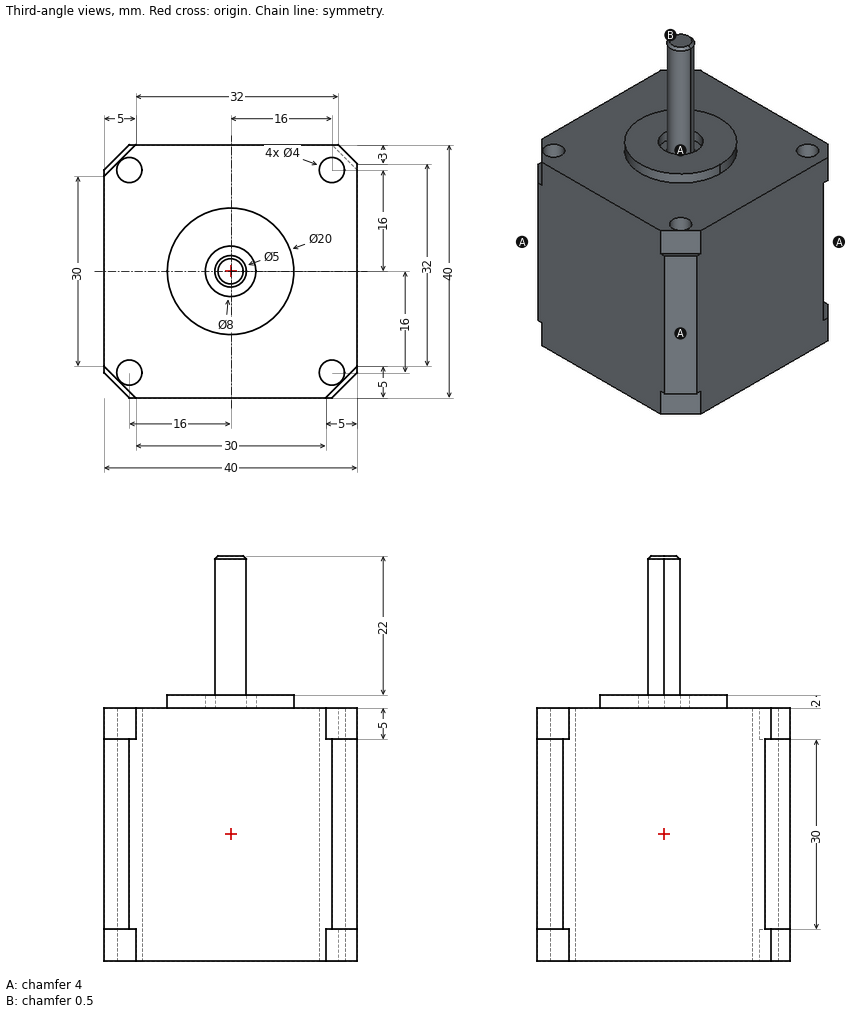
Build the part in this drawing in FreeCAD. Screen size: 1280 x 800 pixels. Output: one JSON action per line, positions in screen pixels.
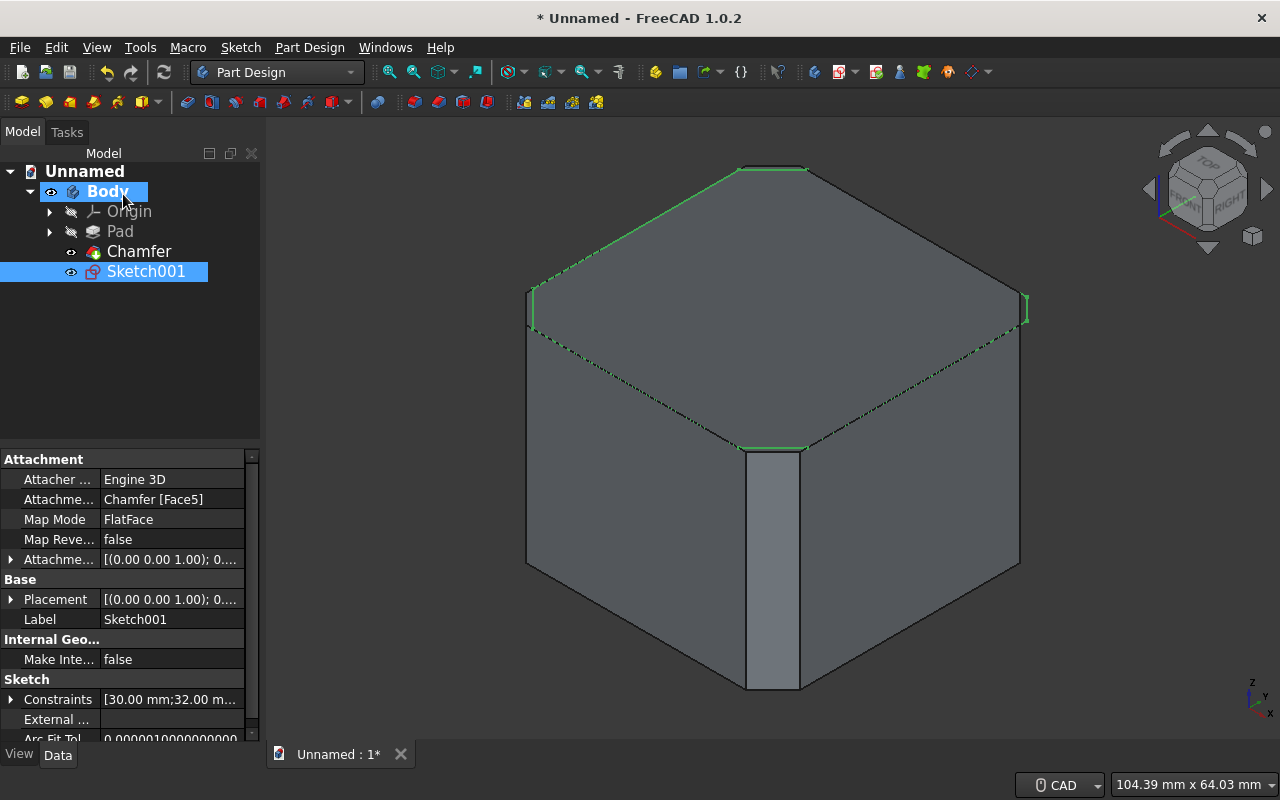
{"action": "left_click", "coordinate": [22, 102]}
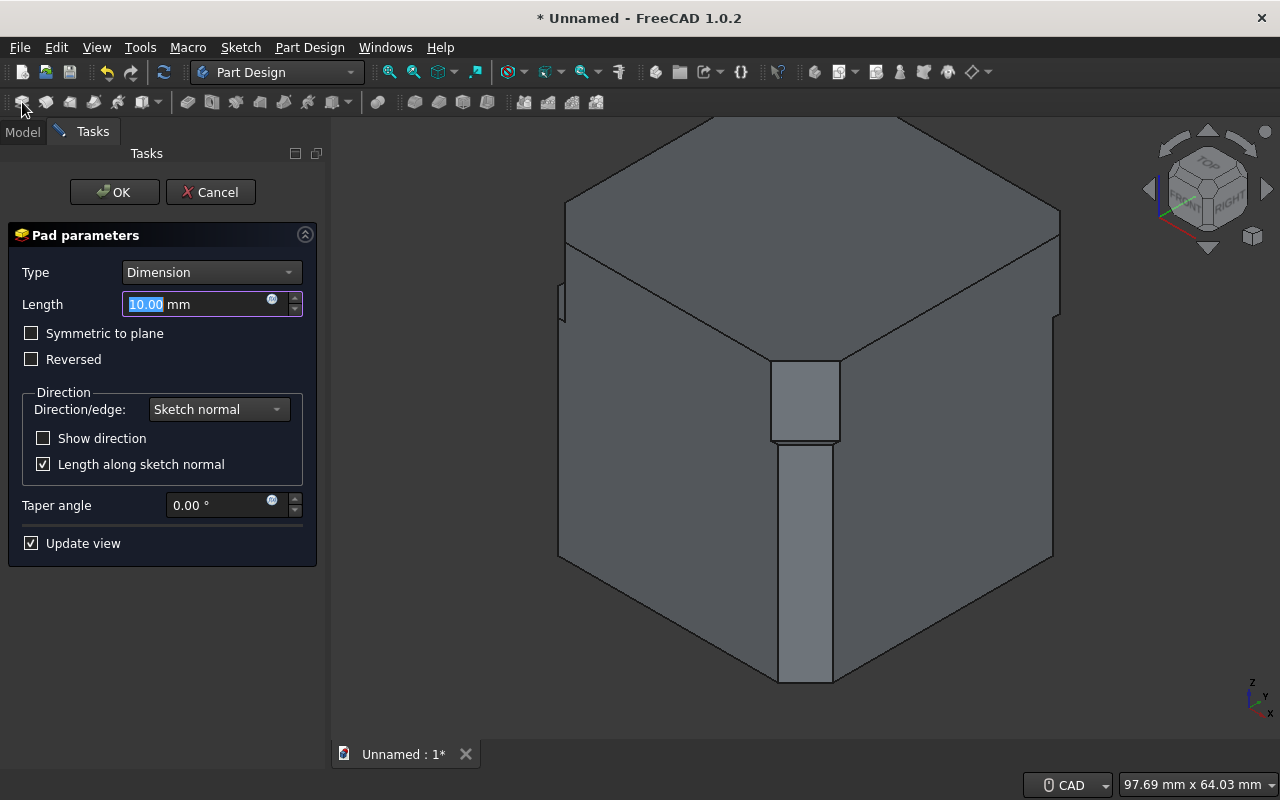
{"action": "type", "text": "5"}
{"action": "key", "text": "Tab"}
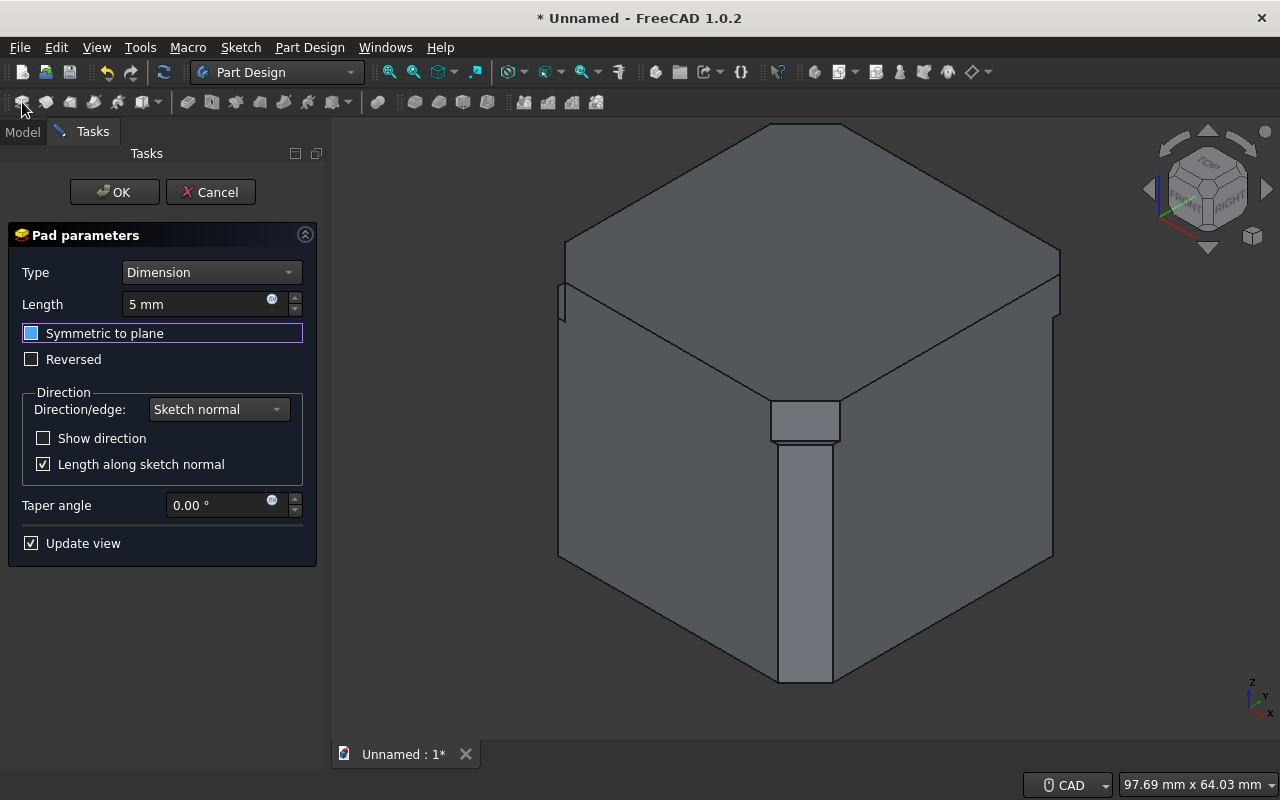
{"action": "left_click", "coordinate": [115, 192]}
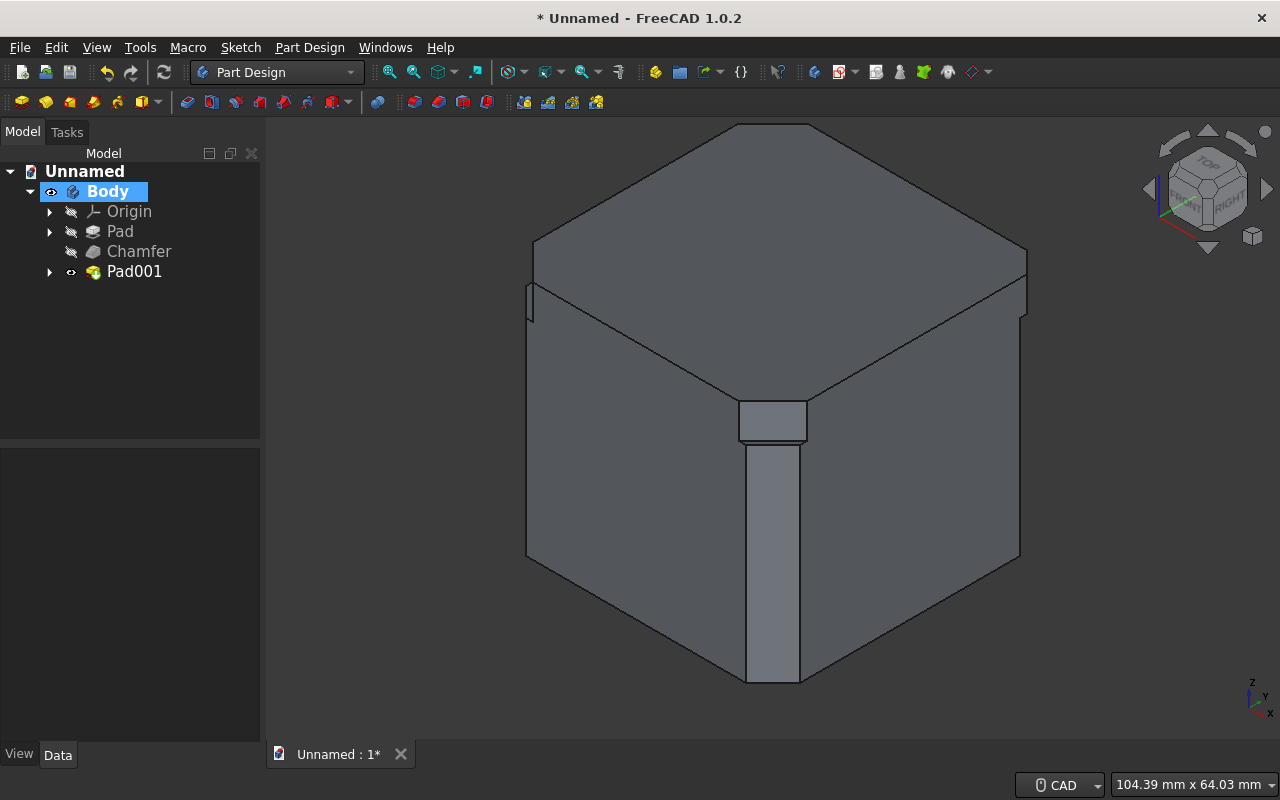
{"action": "left_click", "coordinate": [390, 72]}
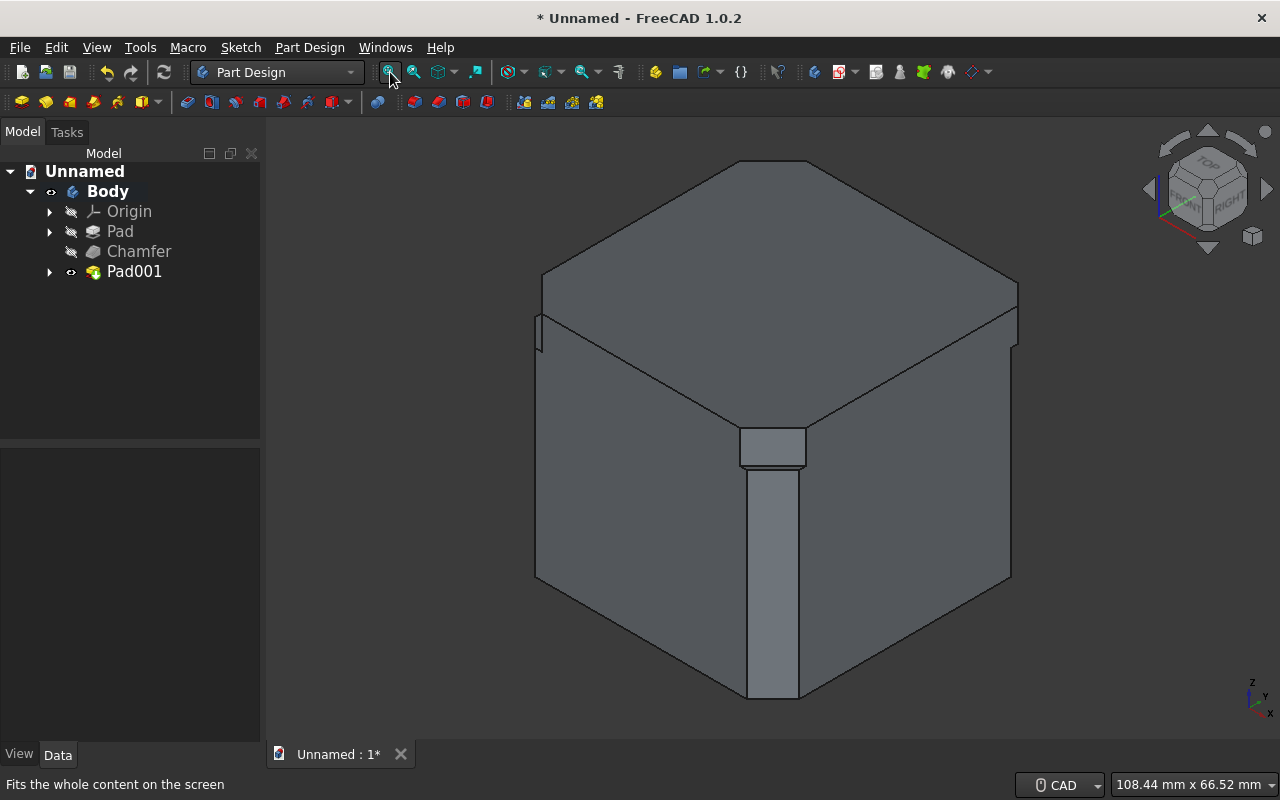
{"action": "left_click", "coordinate": [116, 272]}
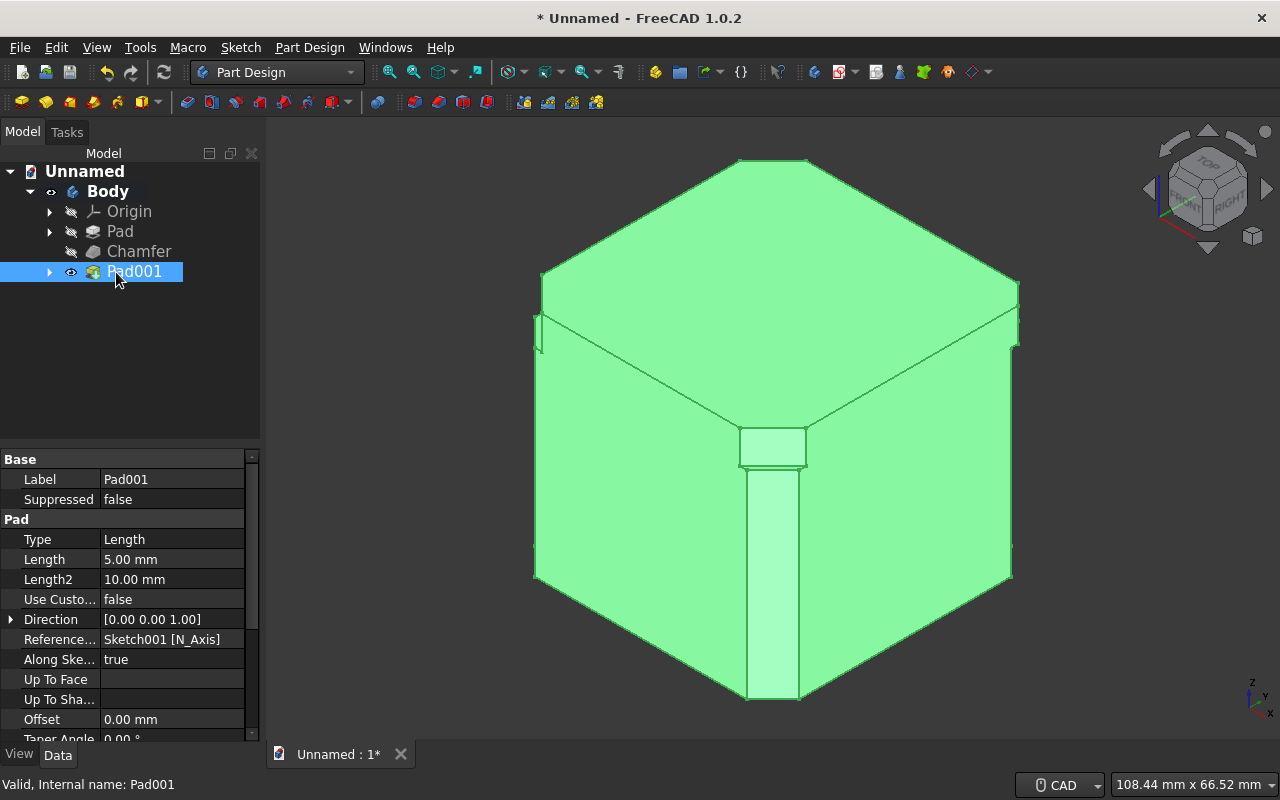
{"action": "left_click", "coordinate": [524, 102]}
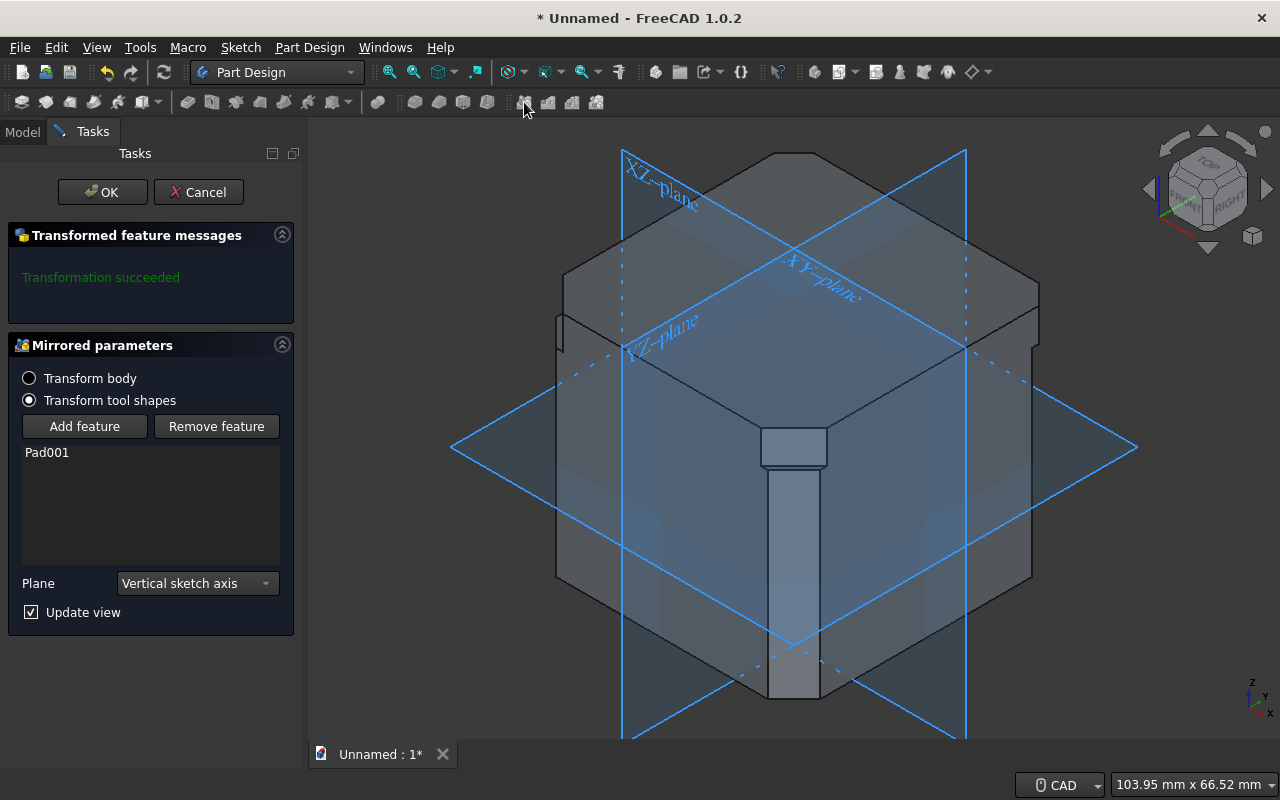
{"action": "left_click", "coordinate": [198, 584]}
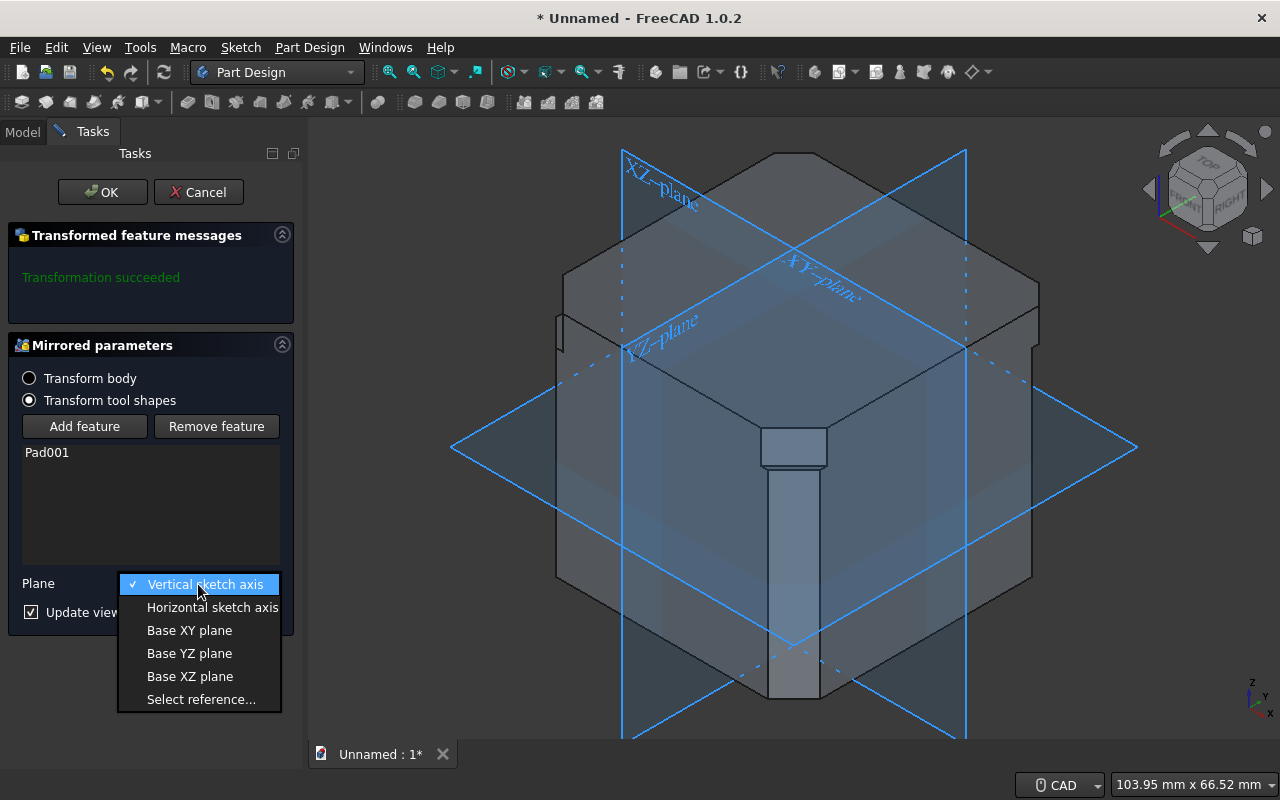
{"action": "left_click", "coordinate": [198, 630]}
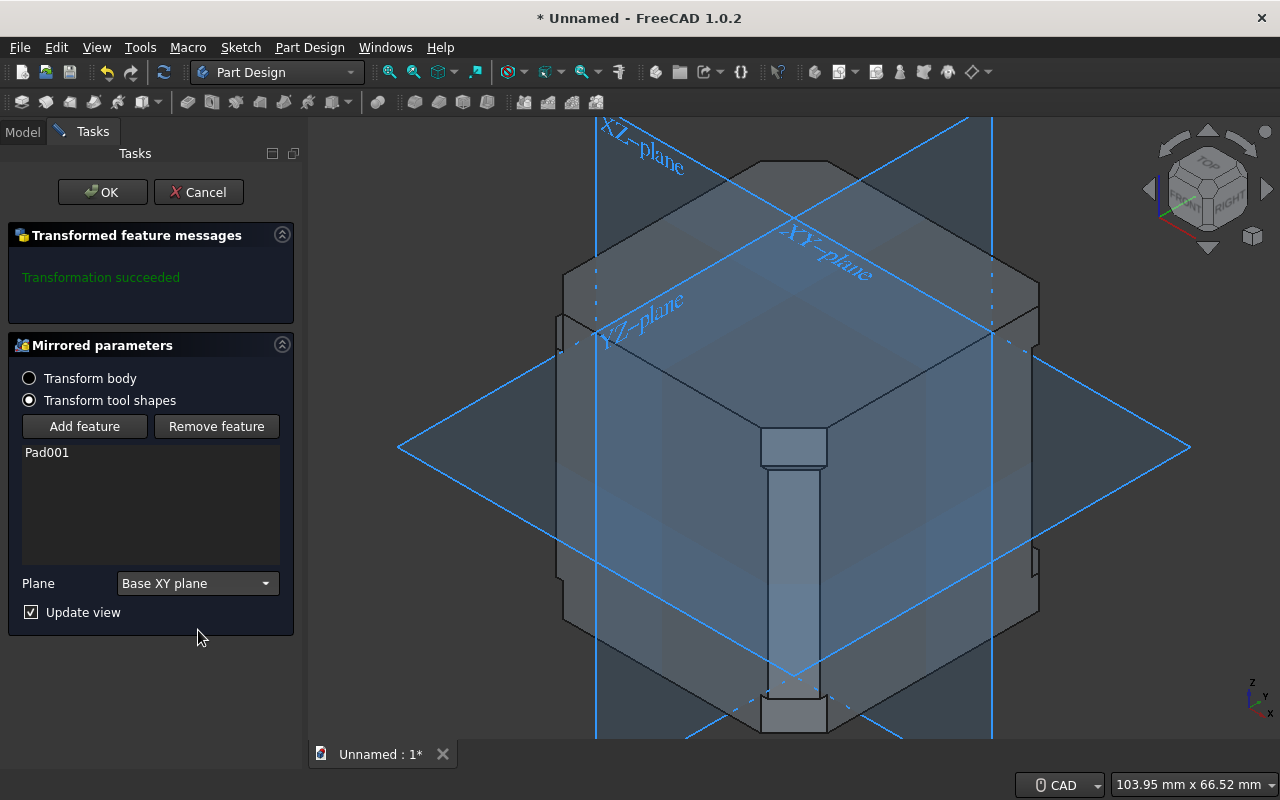
{"action": "left_click", "coordinate": [103, 192]}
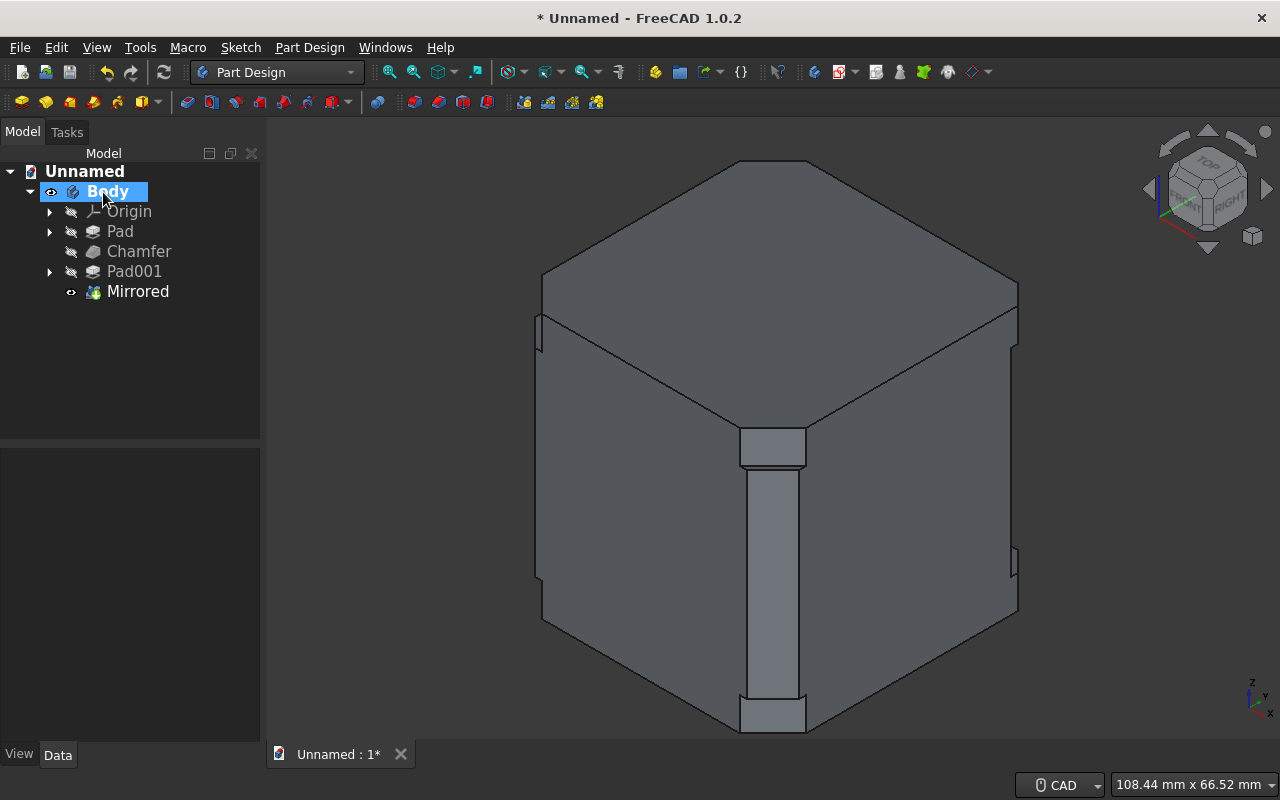
{"action": "left_click", "coordinate": [390, 72]}